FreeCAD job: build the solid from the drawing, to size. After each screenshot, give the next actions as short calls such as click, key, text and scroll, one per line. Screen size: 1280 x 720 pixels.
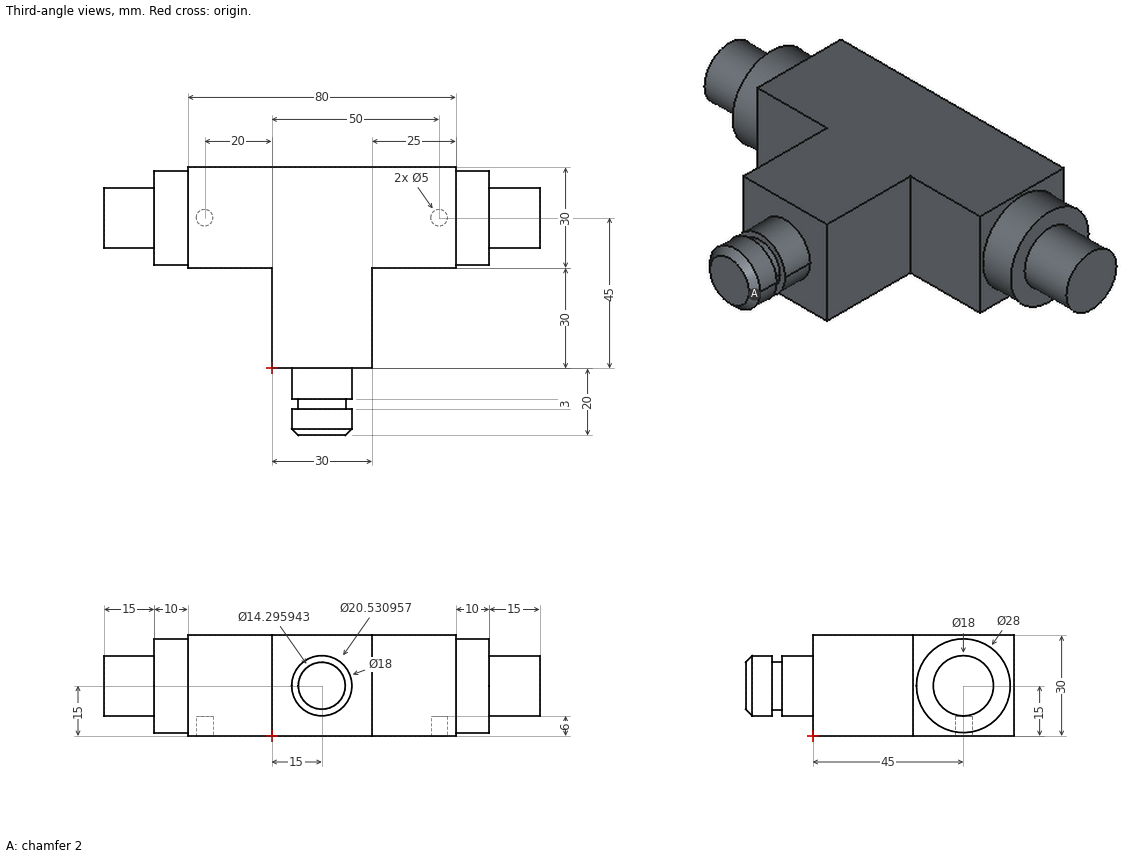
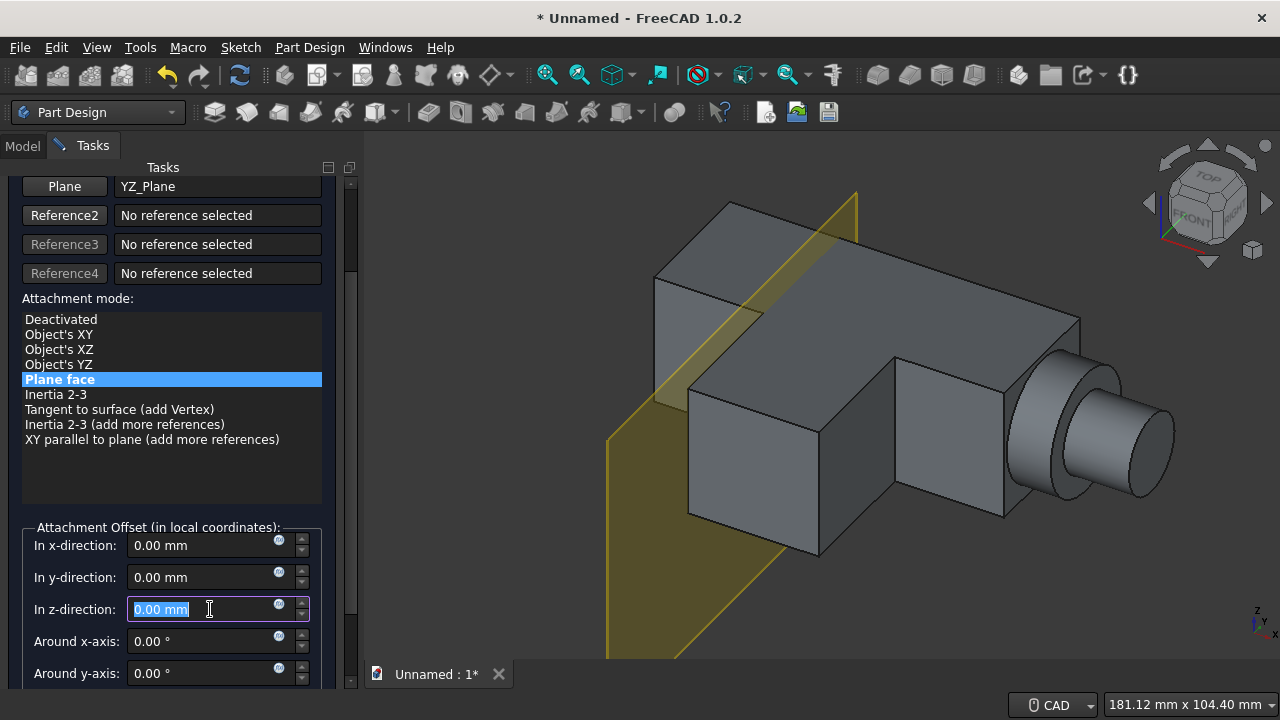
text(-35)
key(Tab)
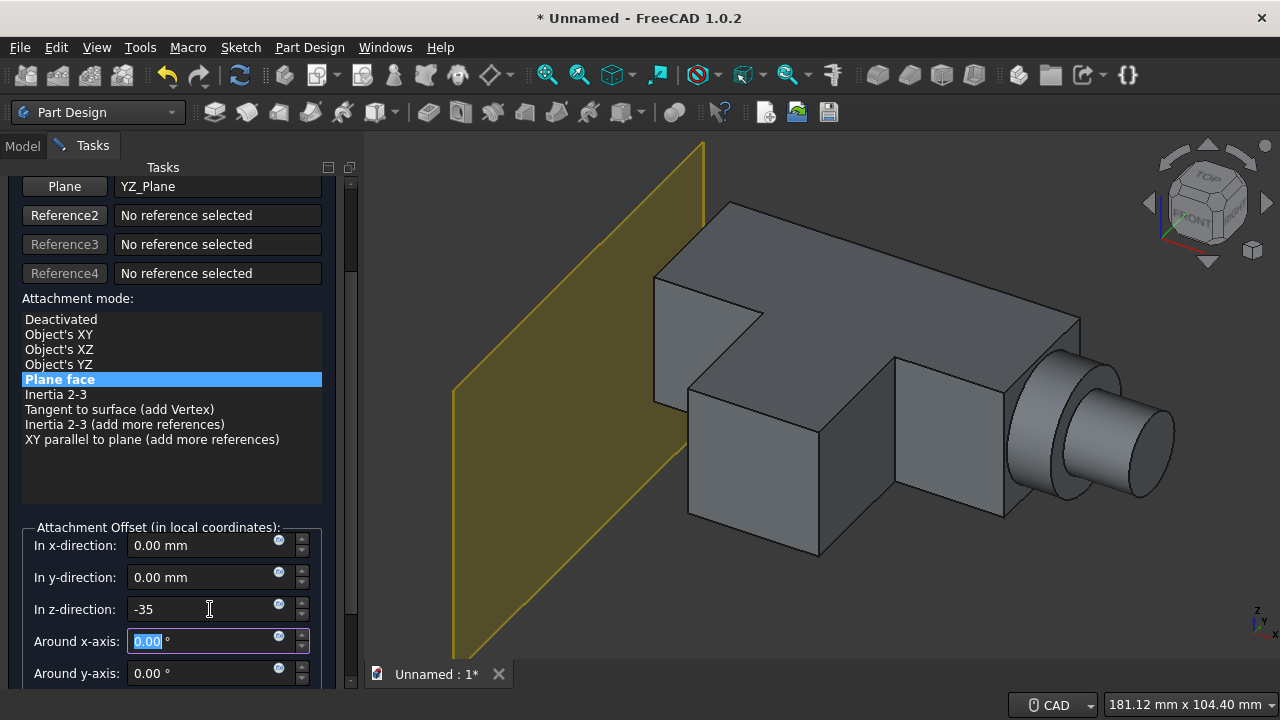
scroll(351, 432, up, 3)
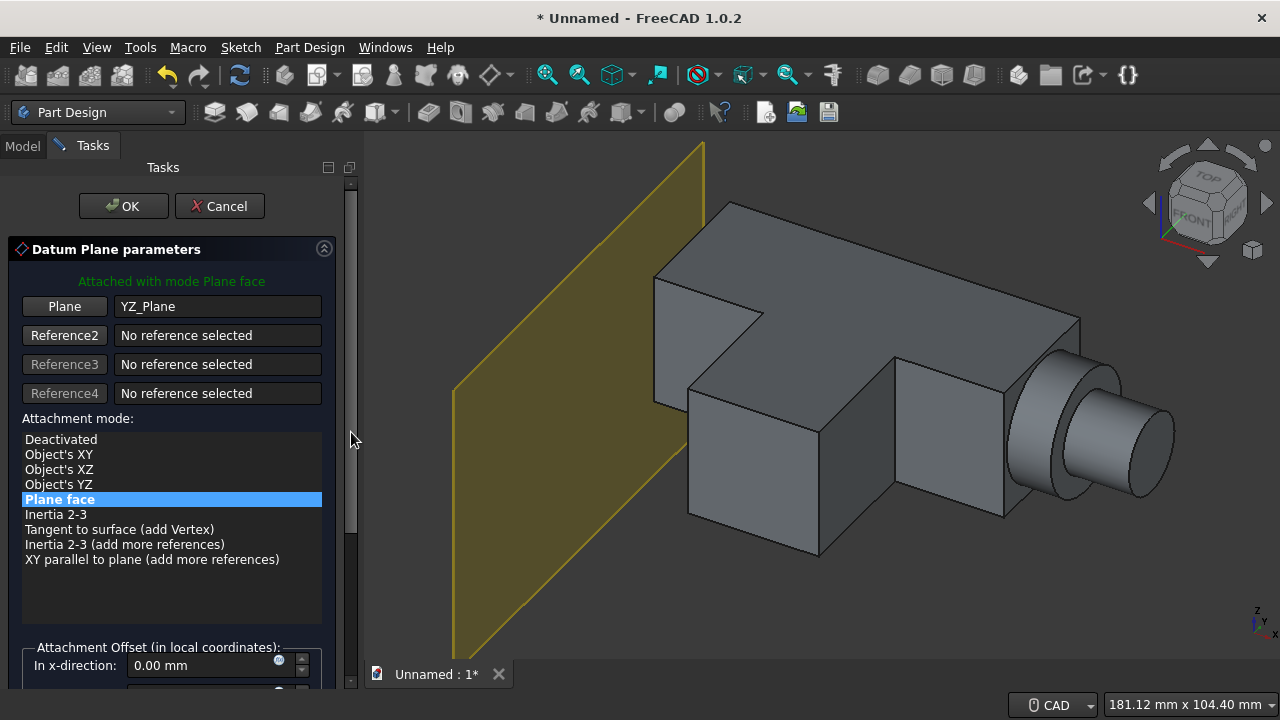
click(124, 206)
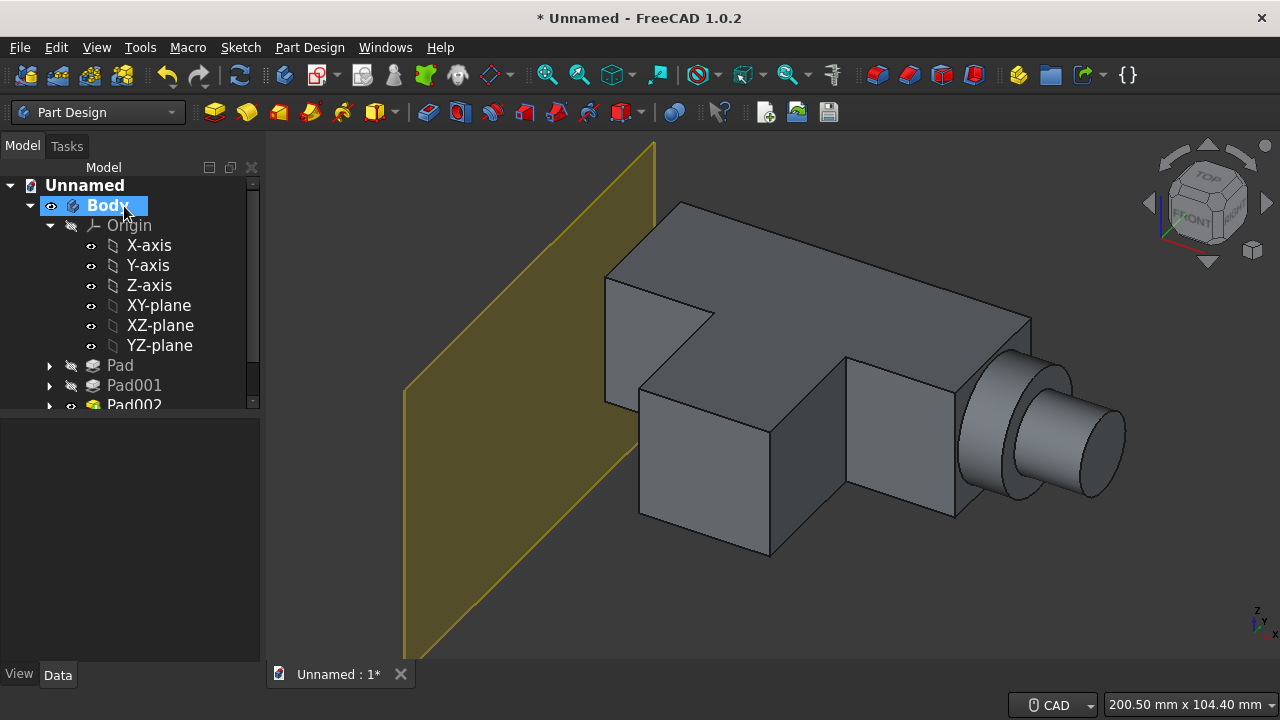
scroll(100, 301, down, 3)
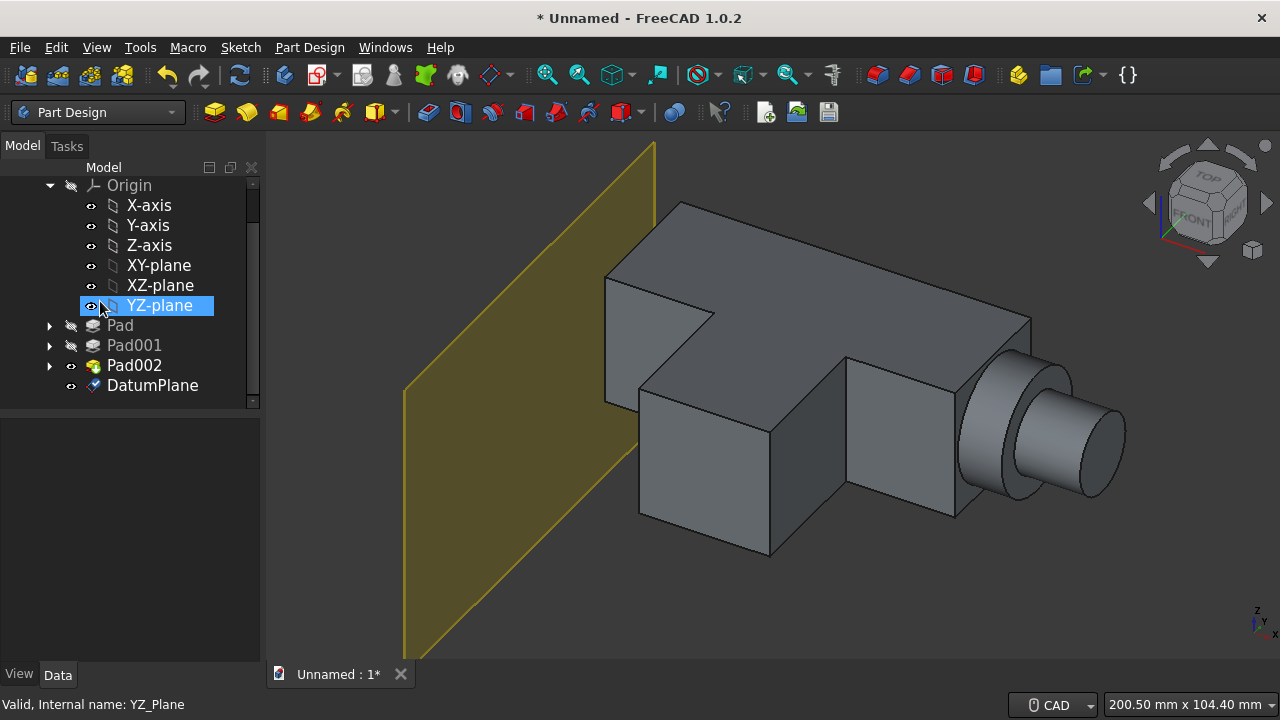
click(116, 386)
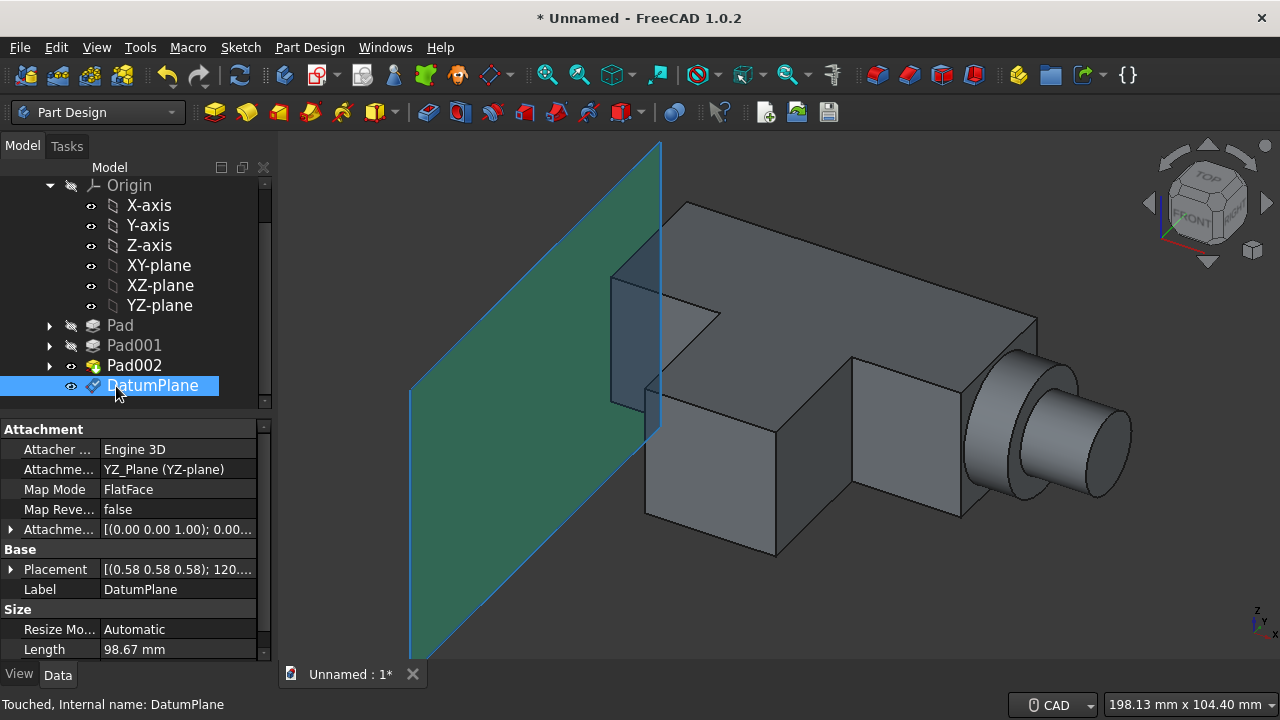
click(318, 76)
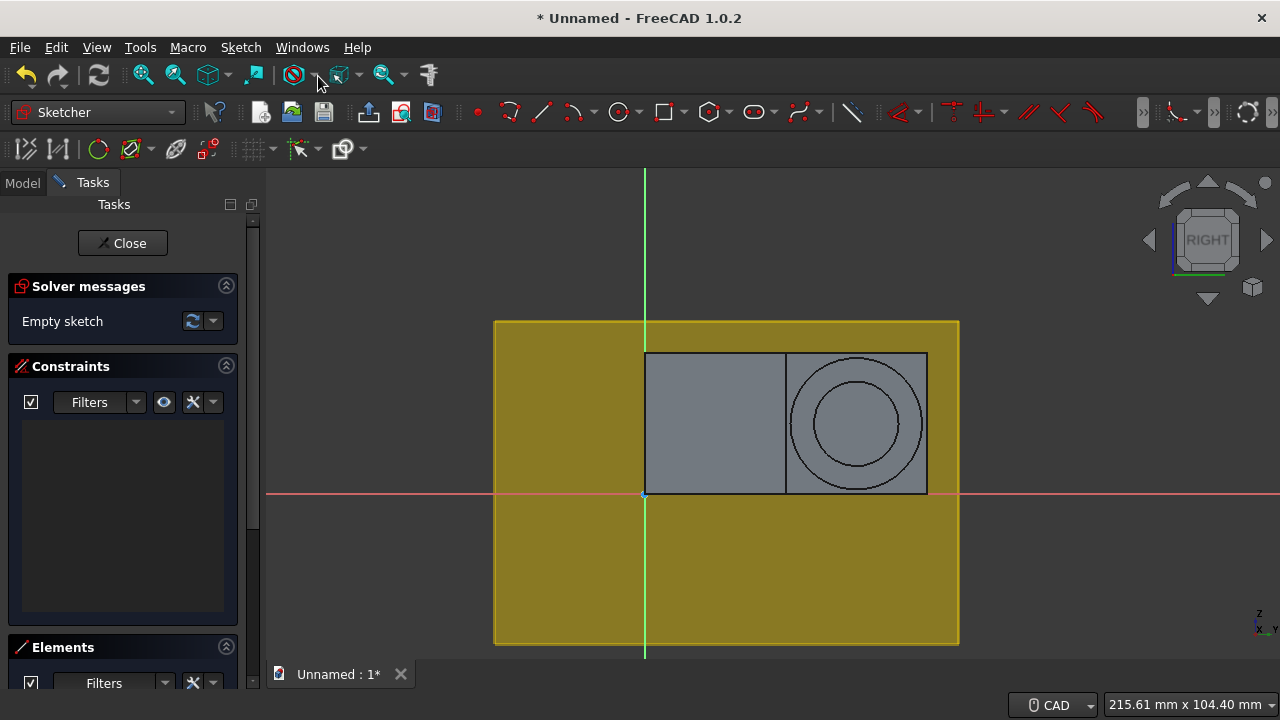
click(434, 112)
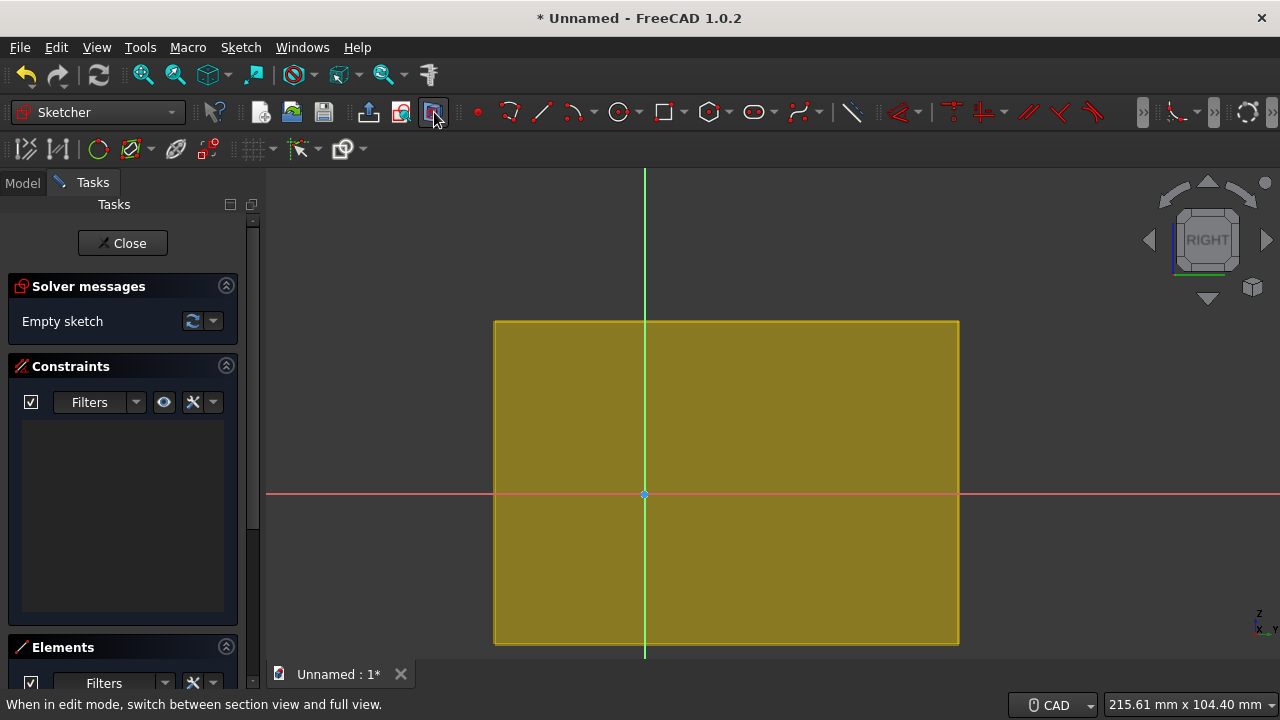
scroll(848, 436, up, 4)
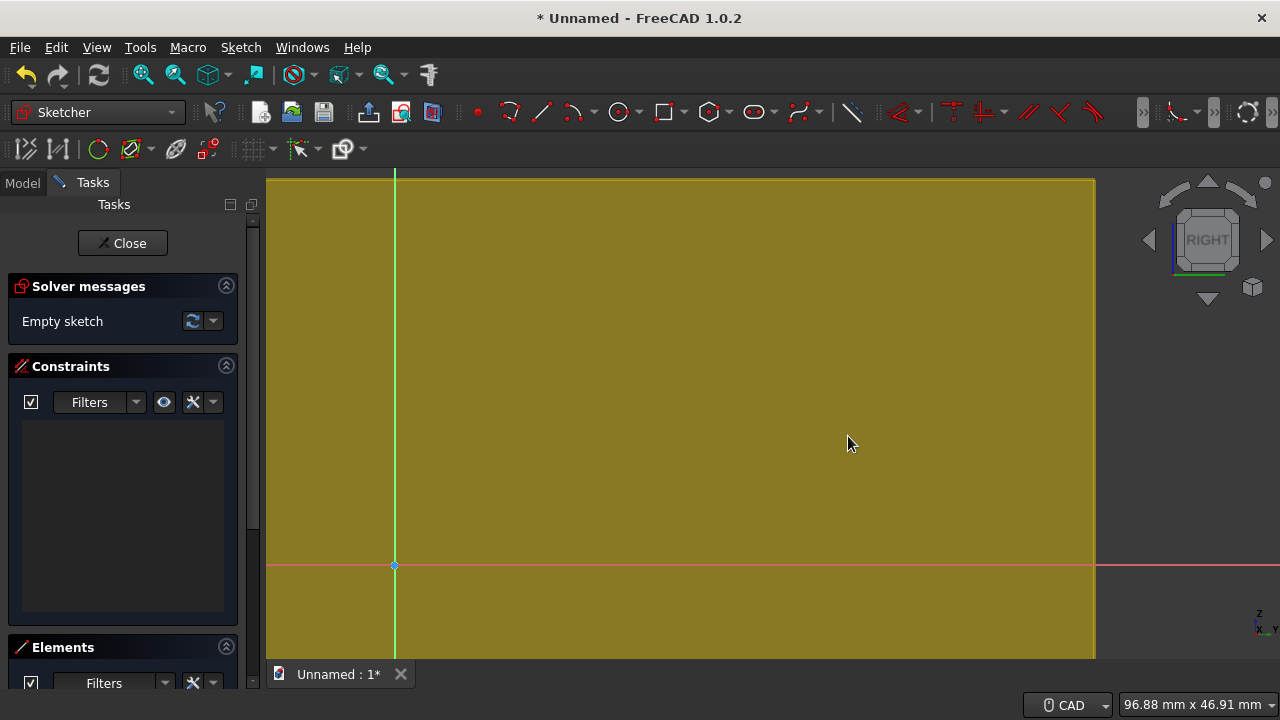
key(g)
key(c)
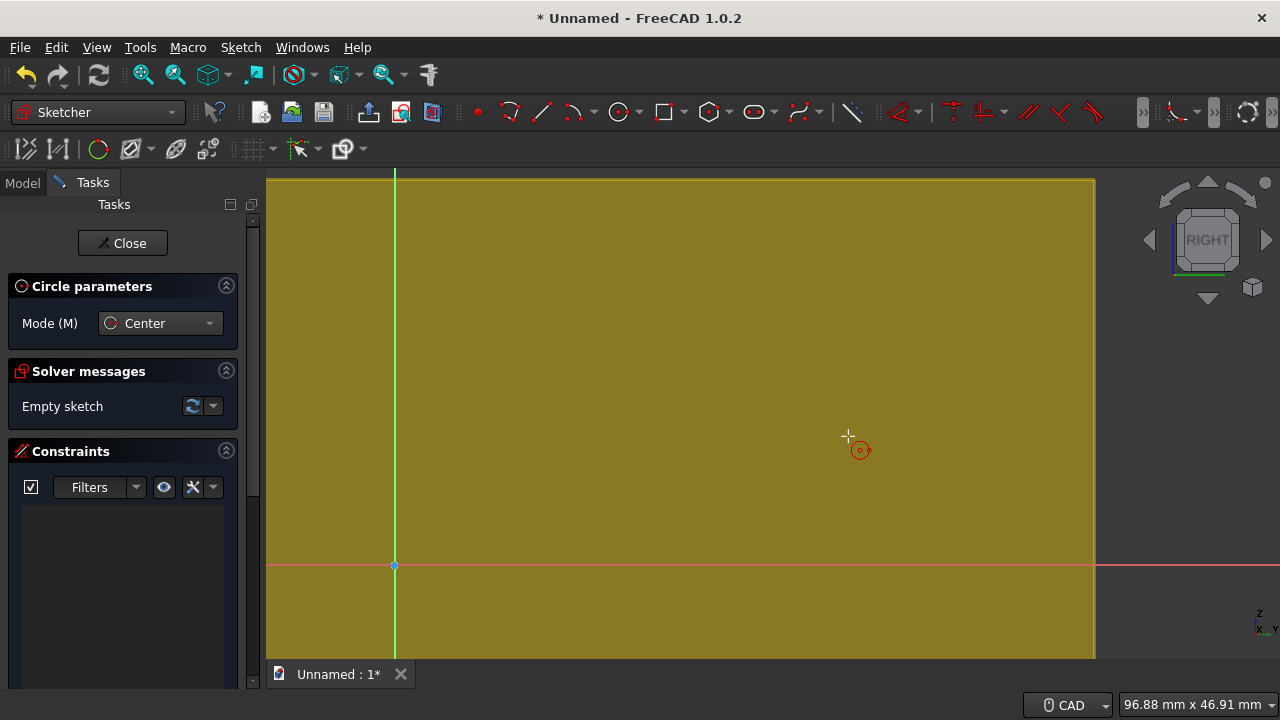
click(866, 408)
move(969, 305)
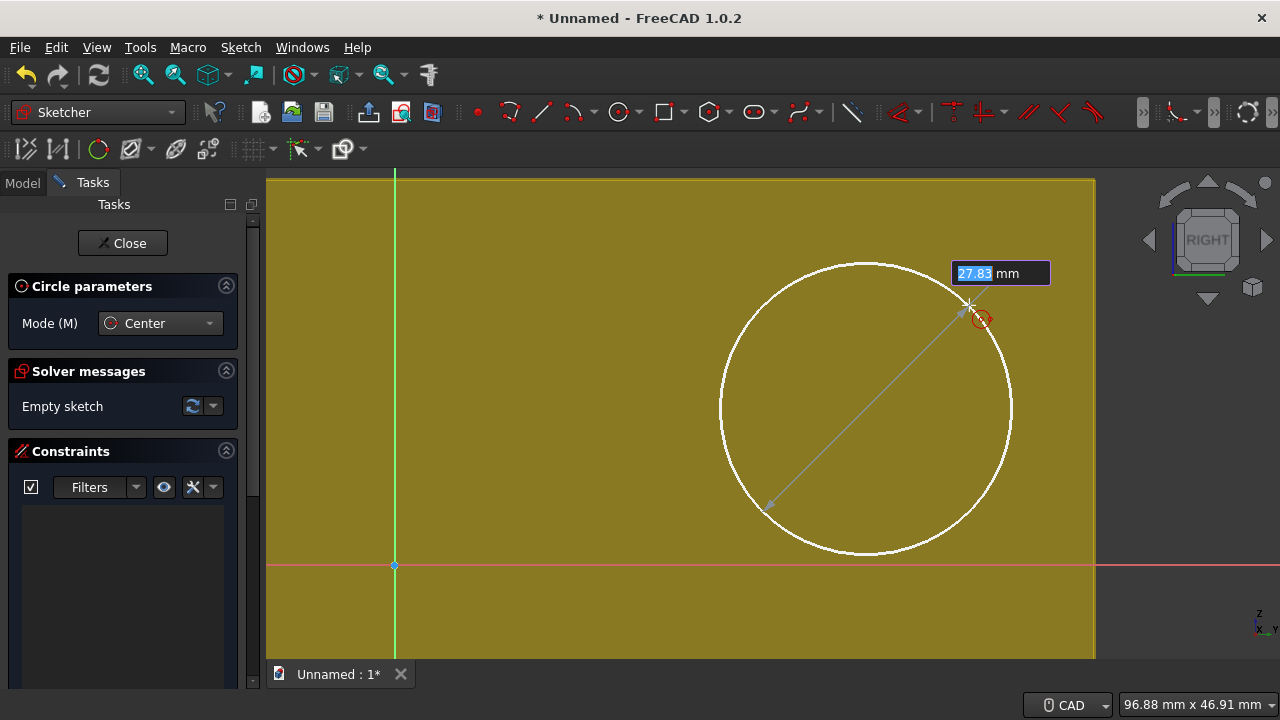
text(28)
key(Return)
key(Escape)